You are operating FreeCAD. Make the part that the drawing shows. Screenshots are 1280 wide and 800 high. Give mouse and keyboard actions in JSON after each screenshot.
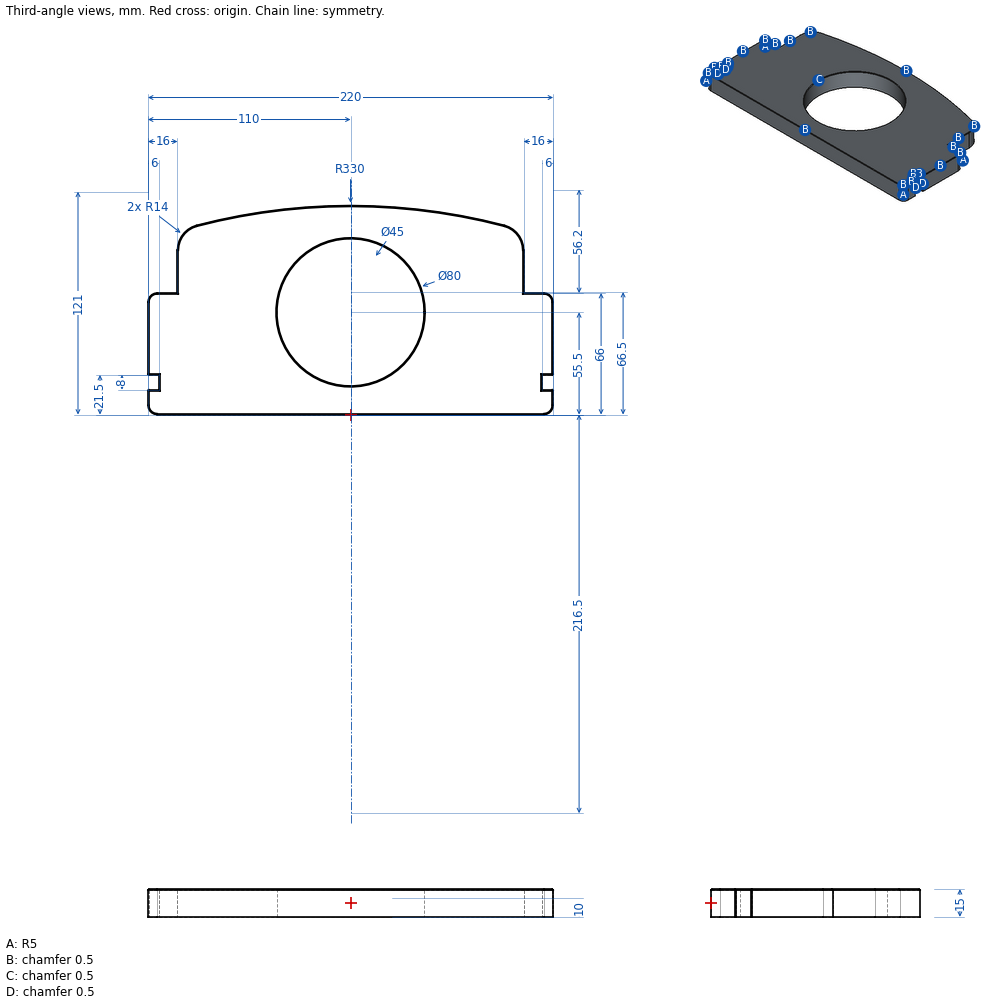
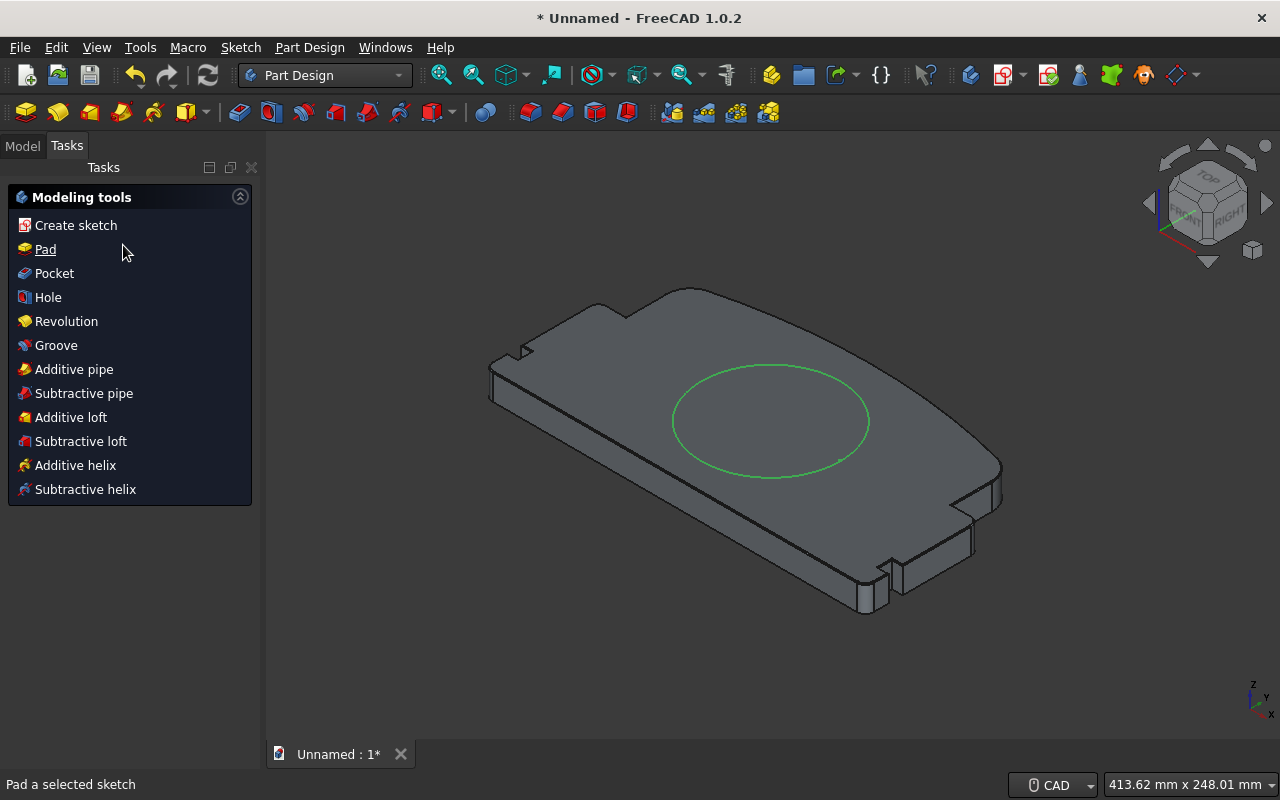
{"action": "left_click", "coordinate": [240, 112]}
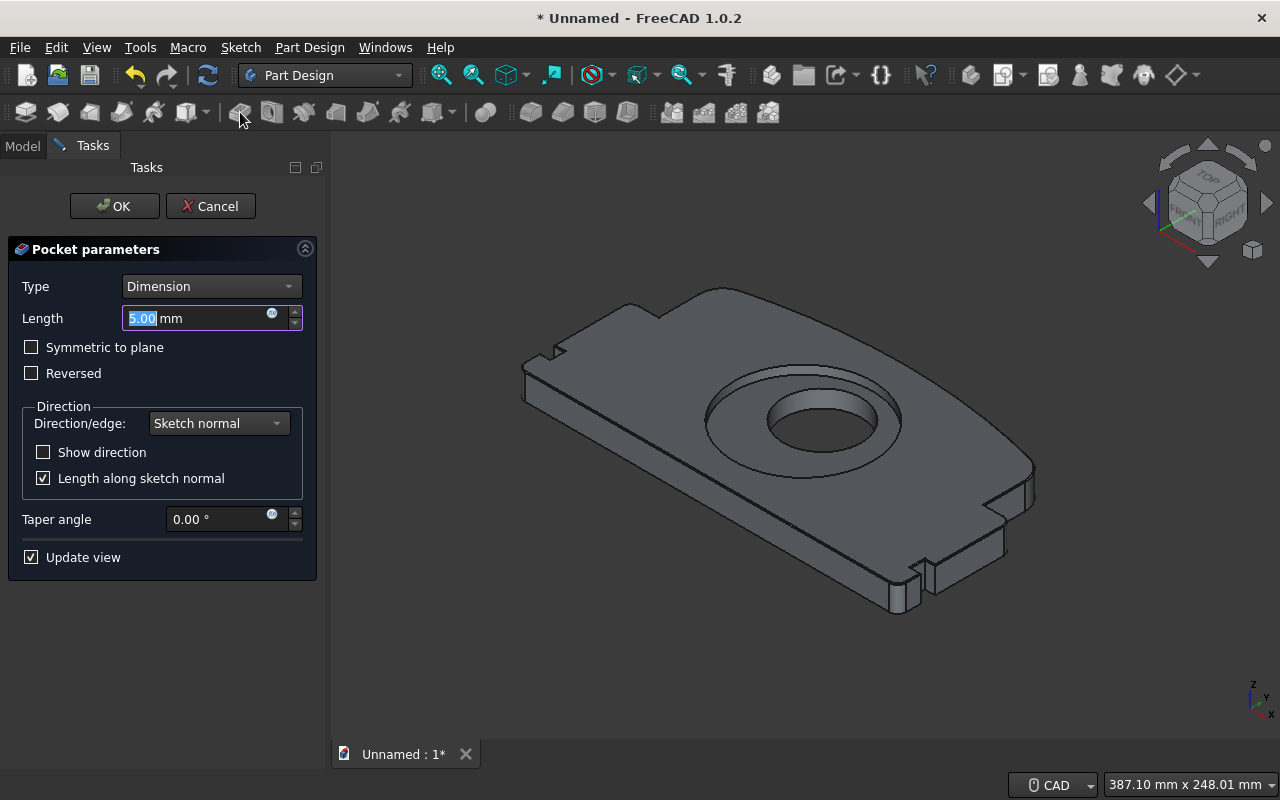
{"action": "left_click", "coordinate": [212, 286]}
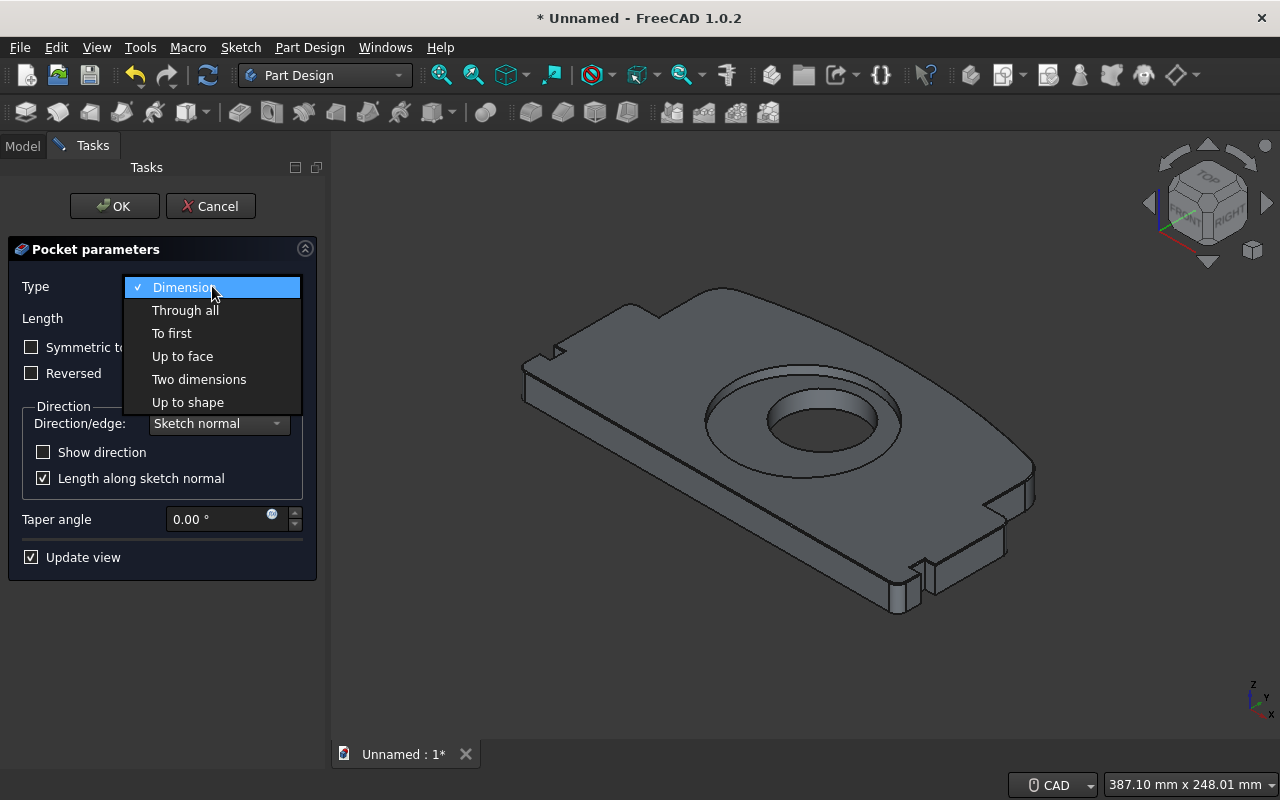
{"action": "left_click", "coordinate": [212, 310]}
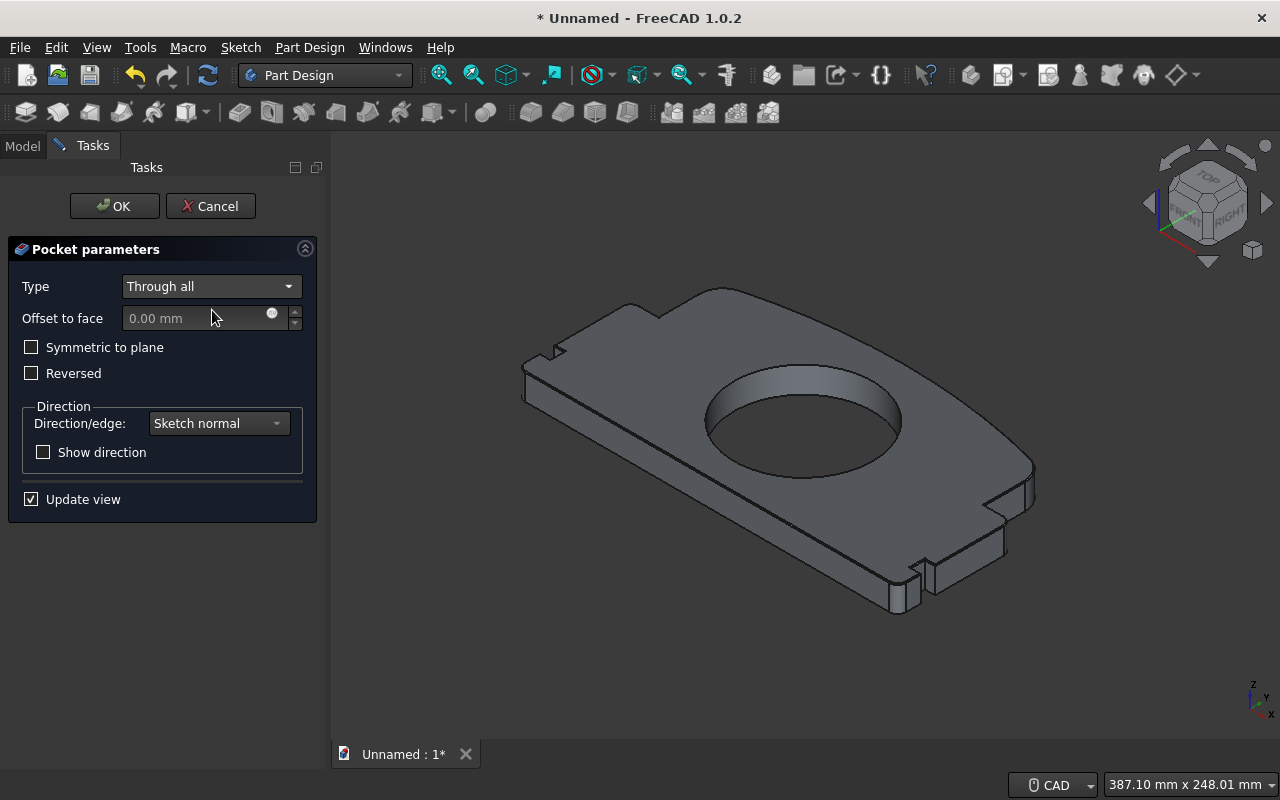
{"action": "left_click", "coordinate": [115, 206]}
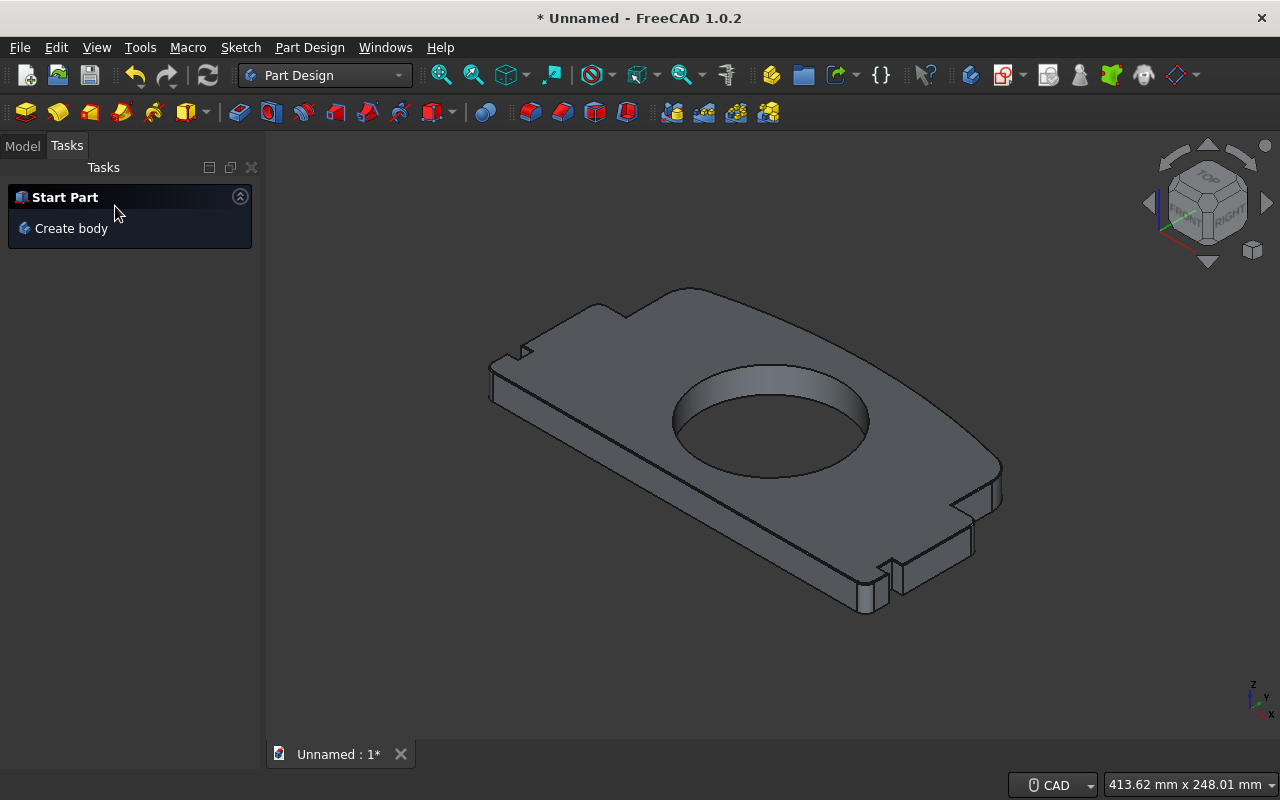
{"action": "left_click", "coordinate": [701, 380]}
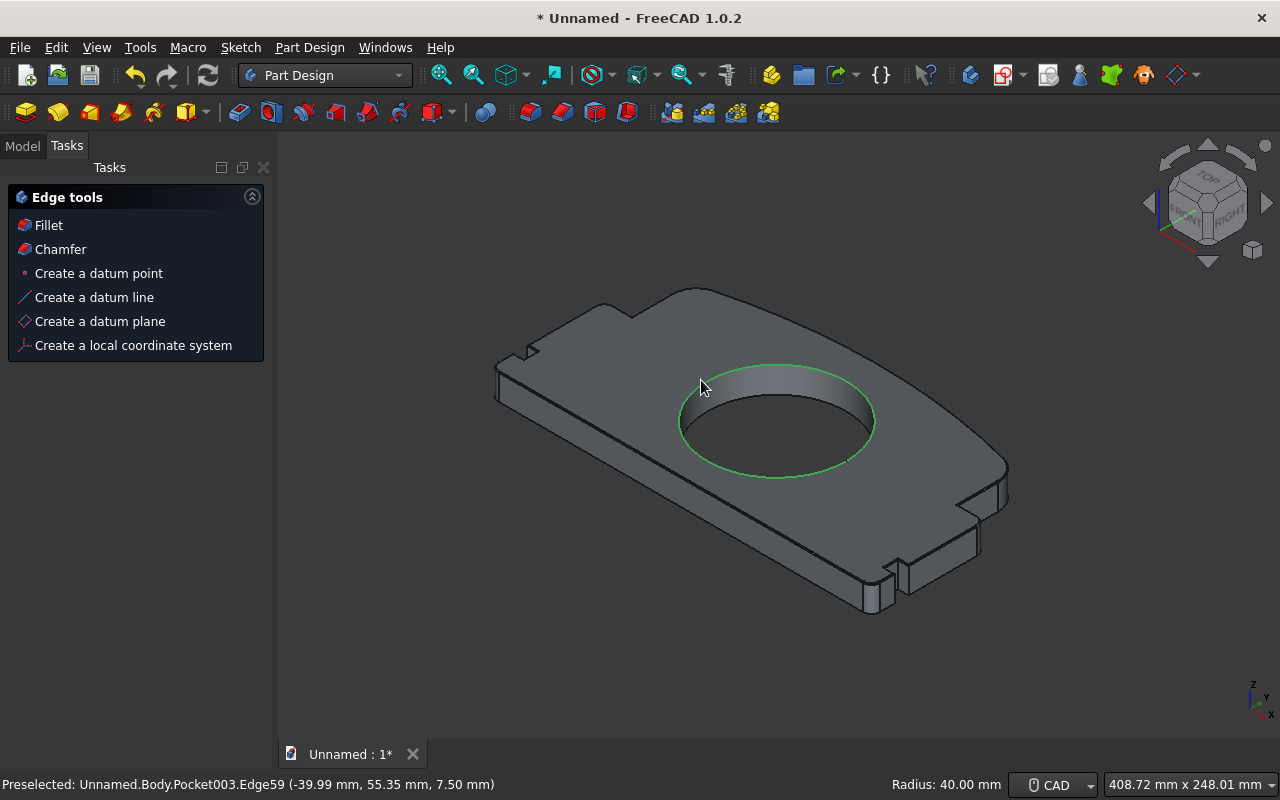
{"action": "left_click", "coordinate": [564, 112]}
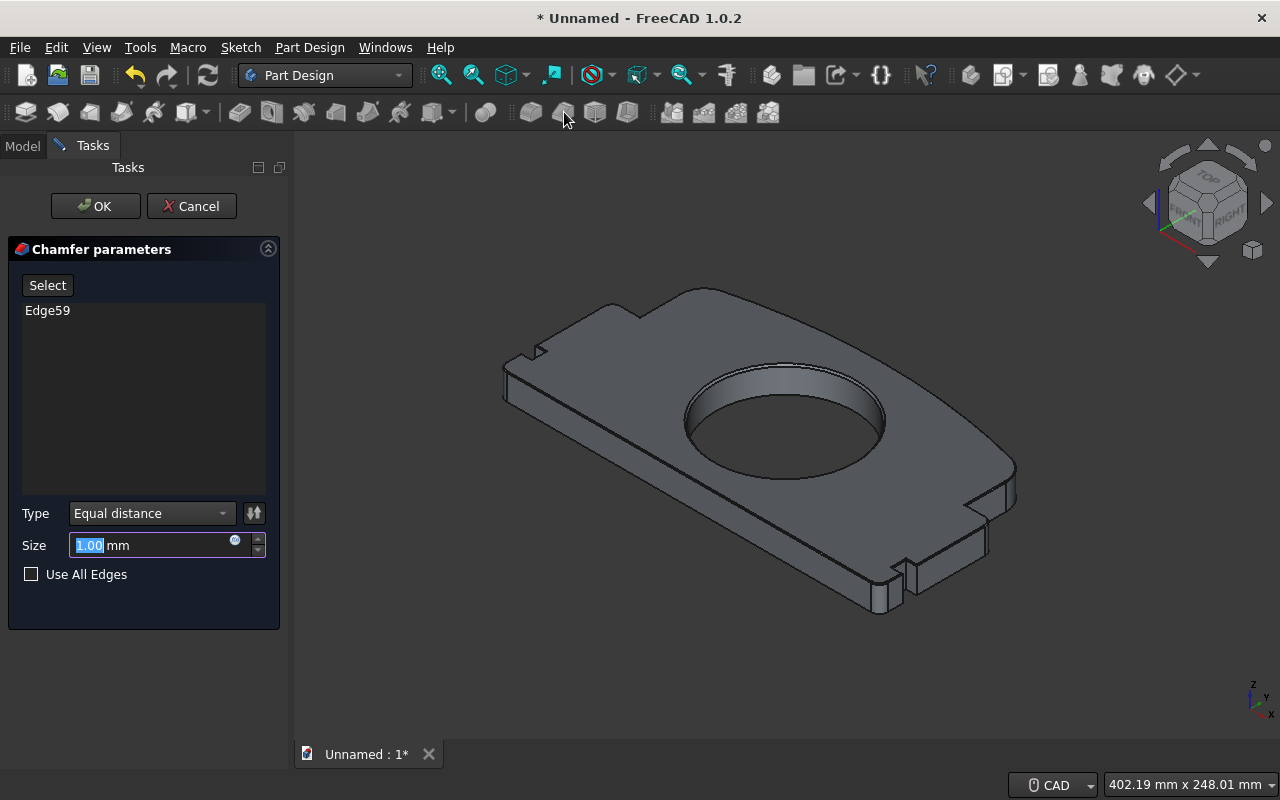
{"action": "type", "text": "0.5"}
{"action": "key", "text": "Tab"}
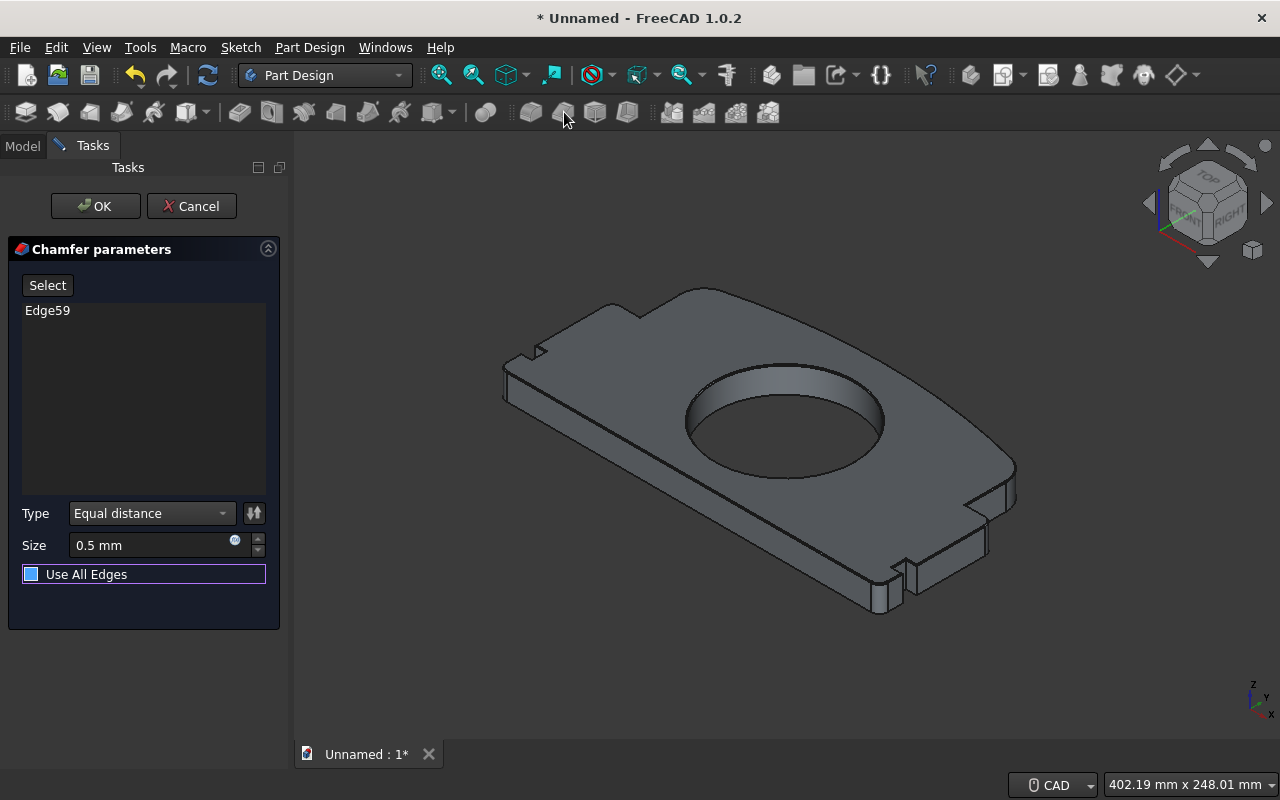
{"action": "left_click", "coordinate": [96, 206]}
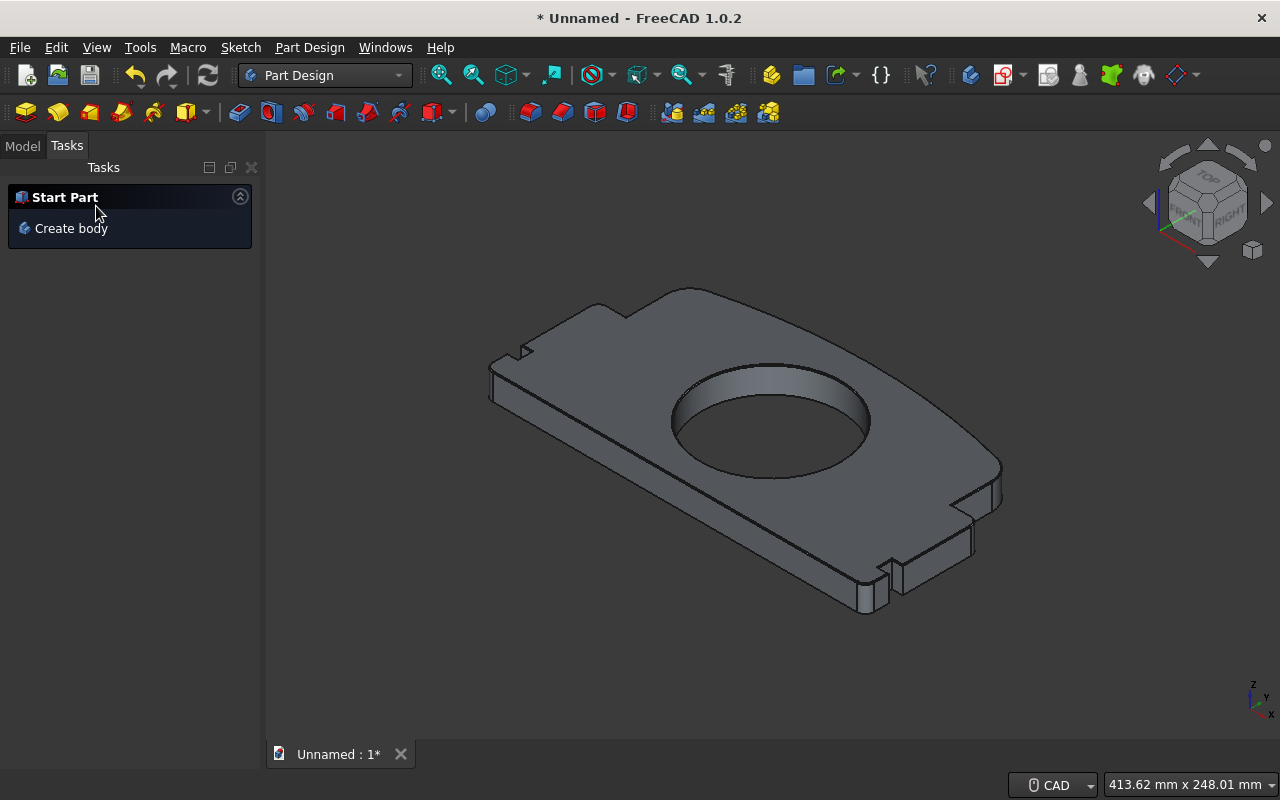
{"action": "left_click", "coordinate": [903, 580]}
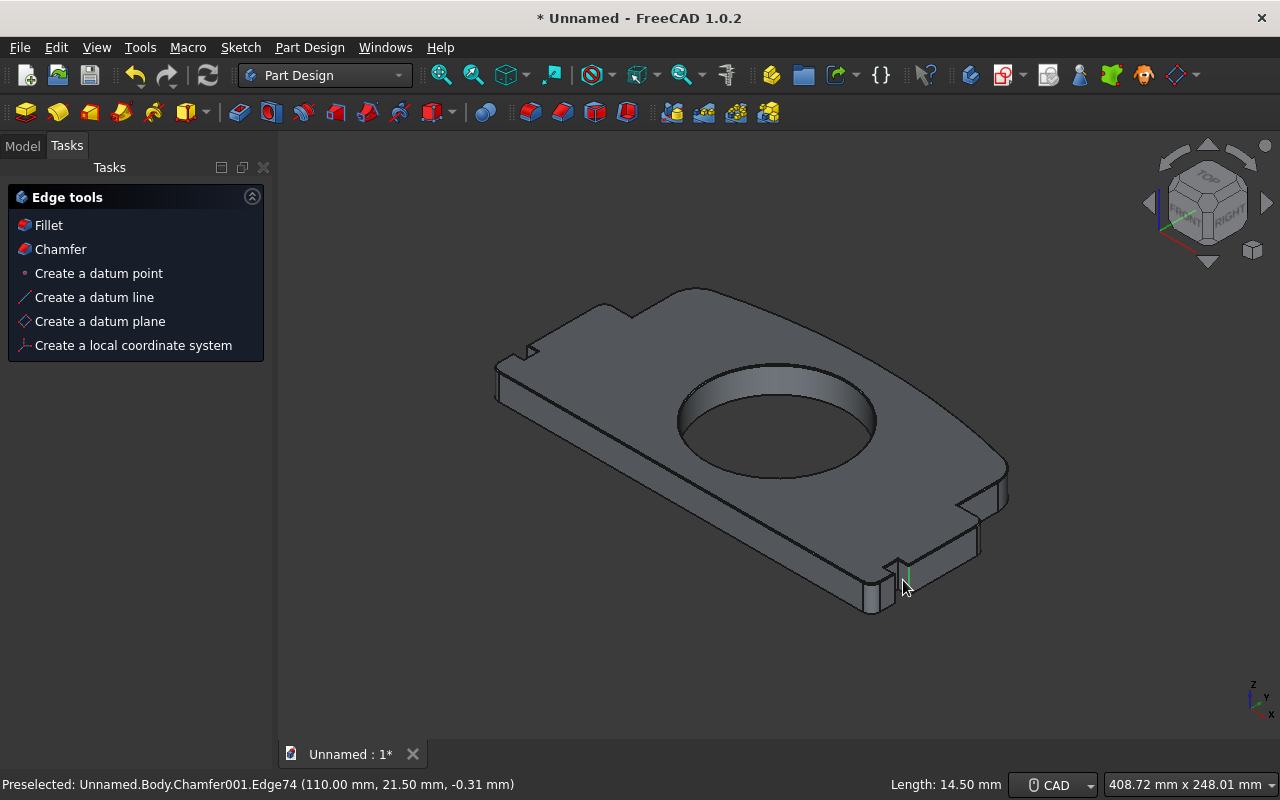
{"action": "key", "text": "2"}